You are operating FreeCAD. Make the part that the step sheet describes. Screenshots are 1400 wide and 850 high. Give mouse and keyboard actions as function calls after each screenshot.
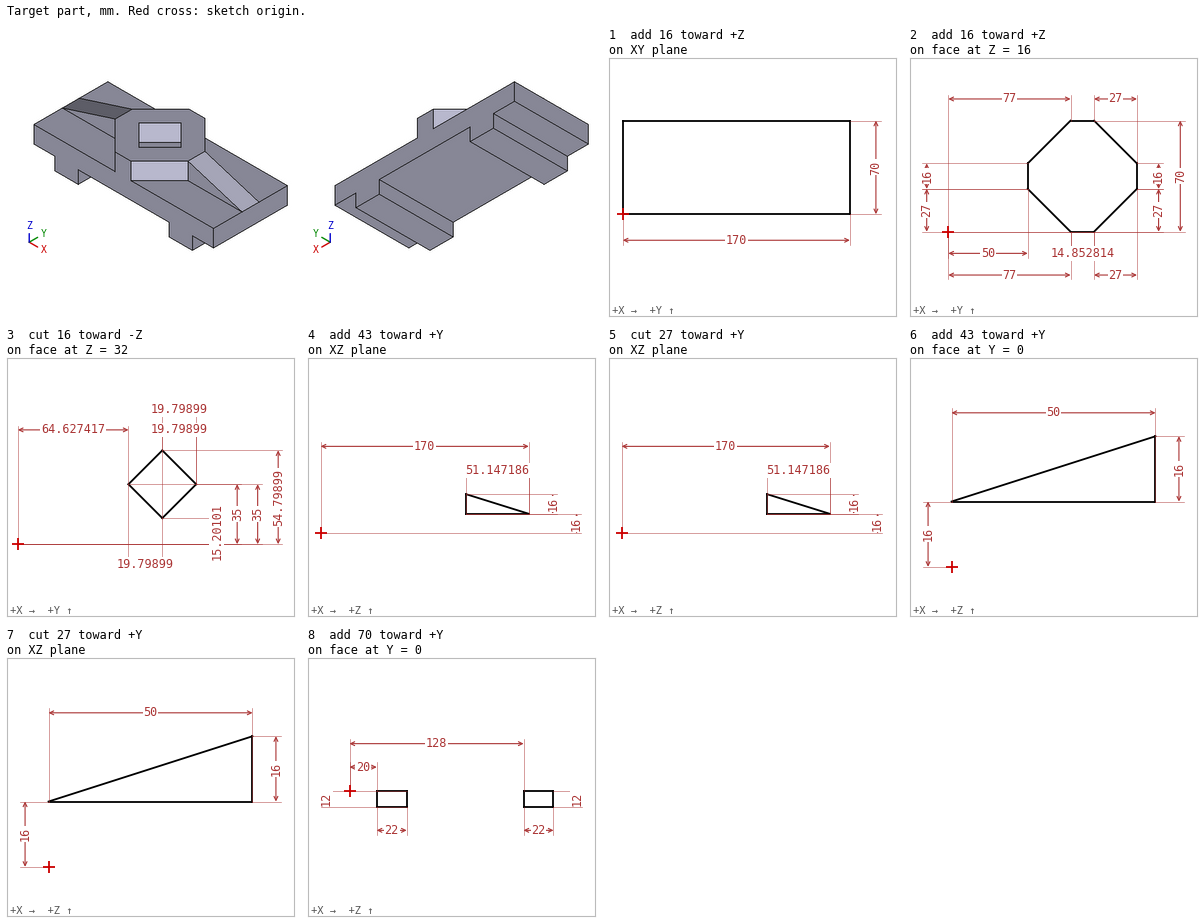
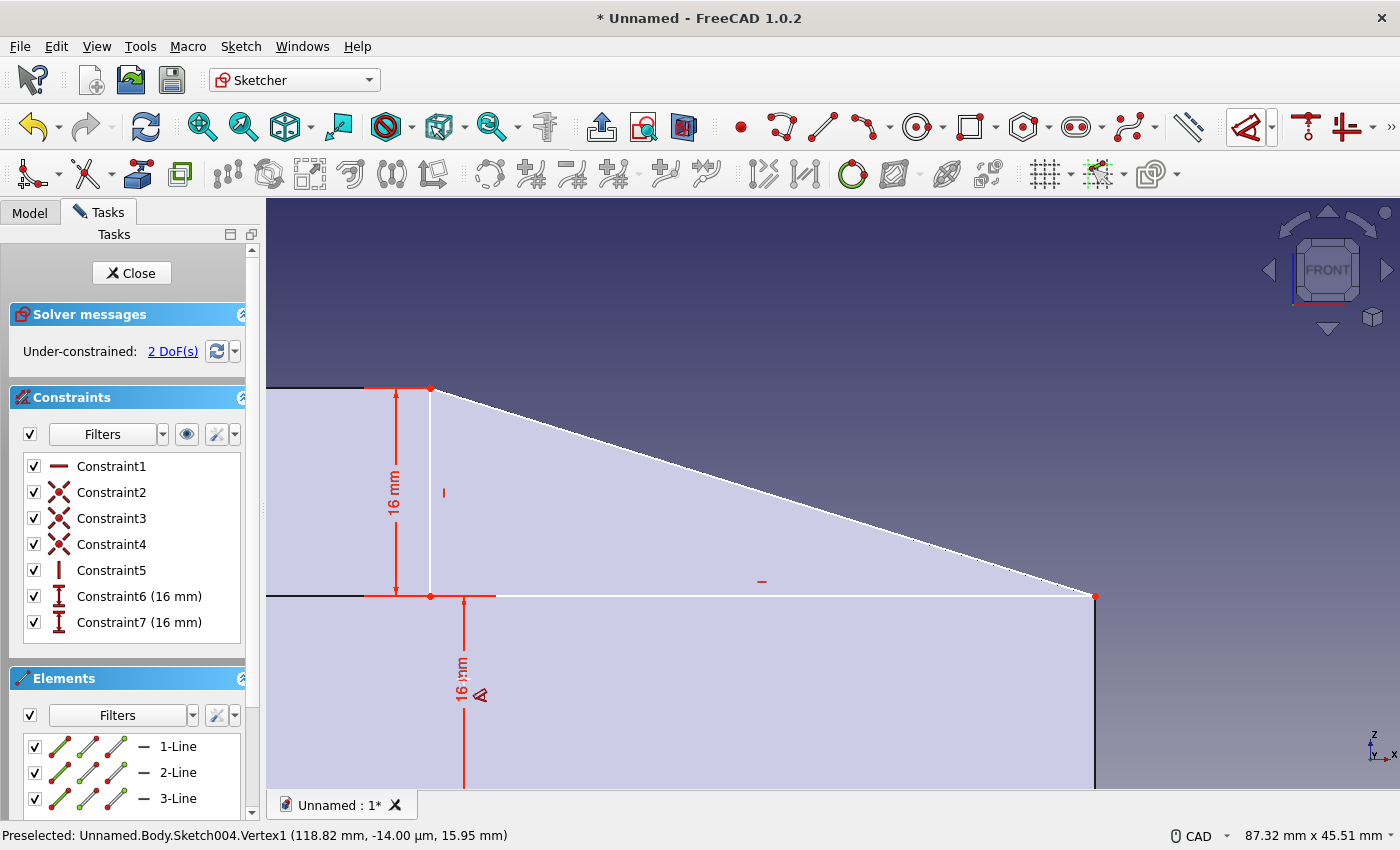
click(1095, 596)
click(695, 562)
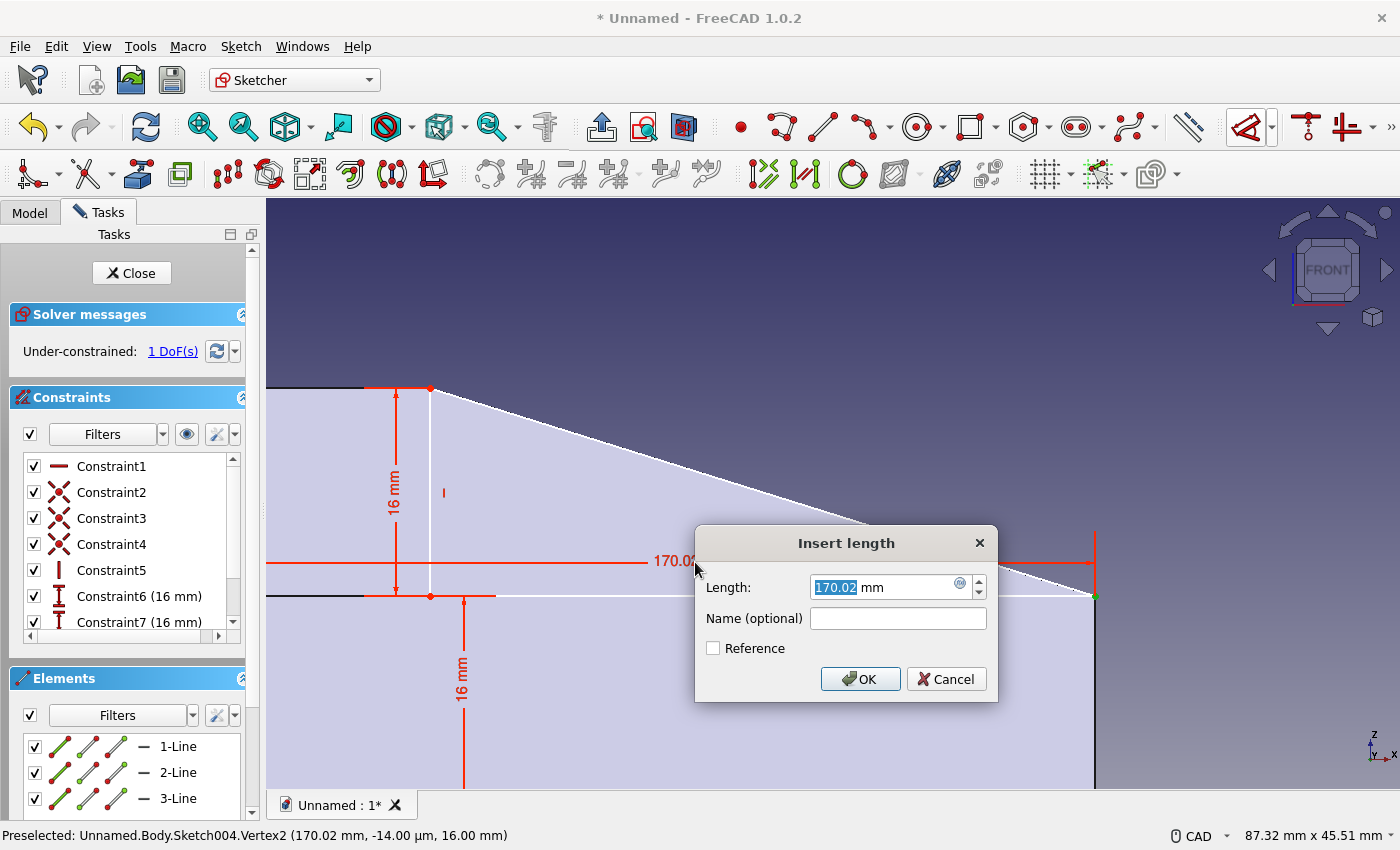
text(170)
key(Return)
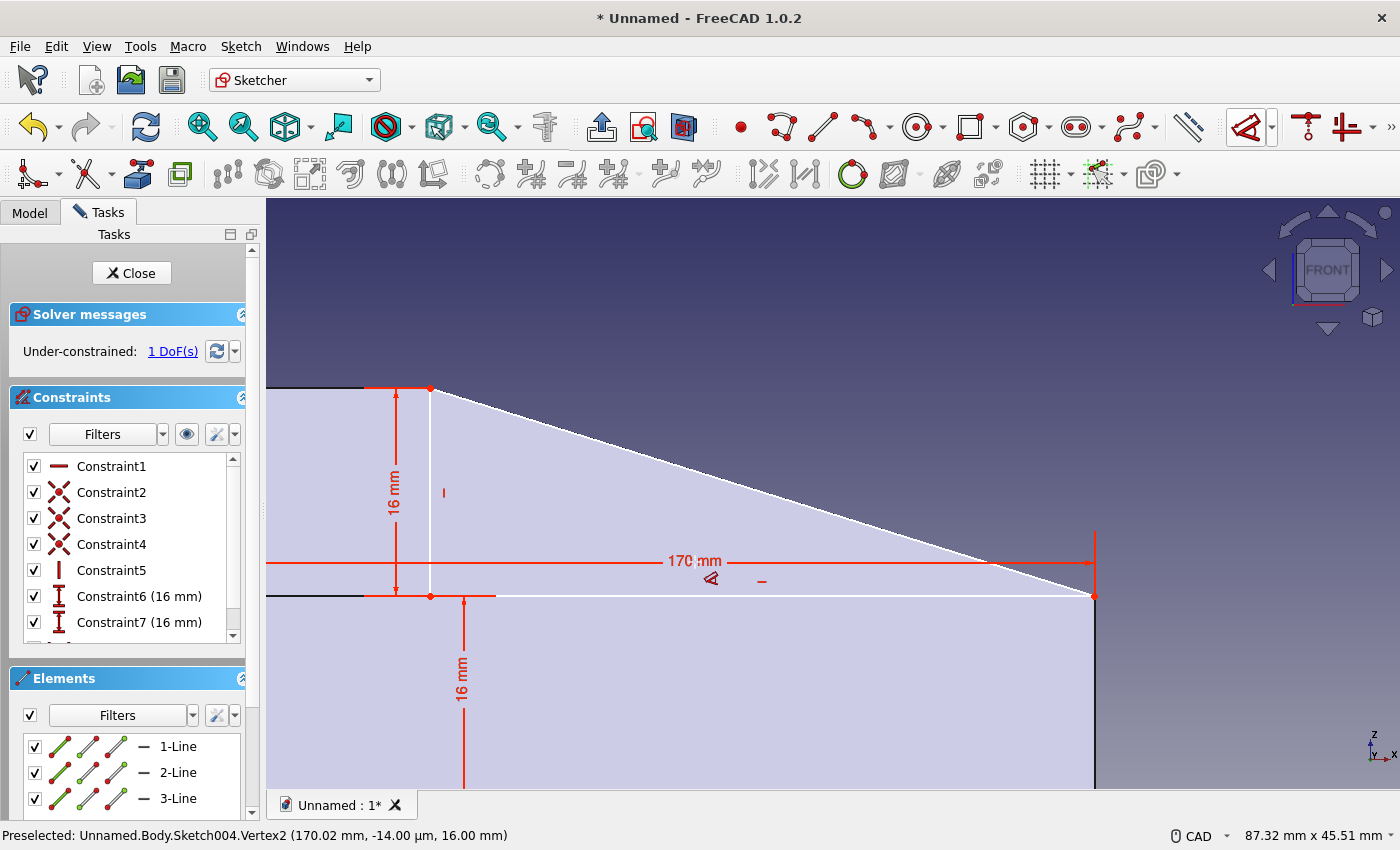
click(629, 596)
click(762, 630)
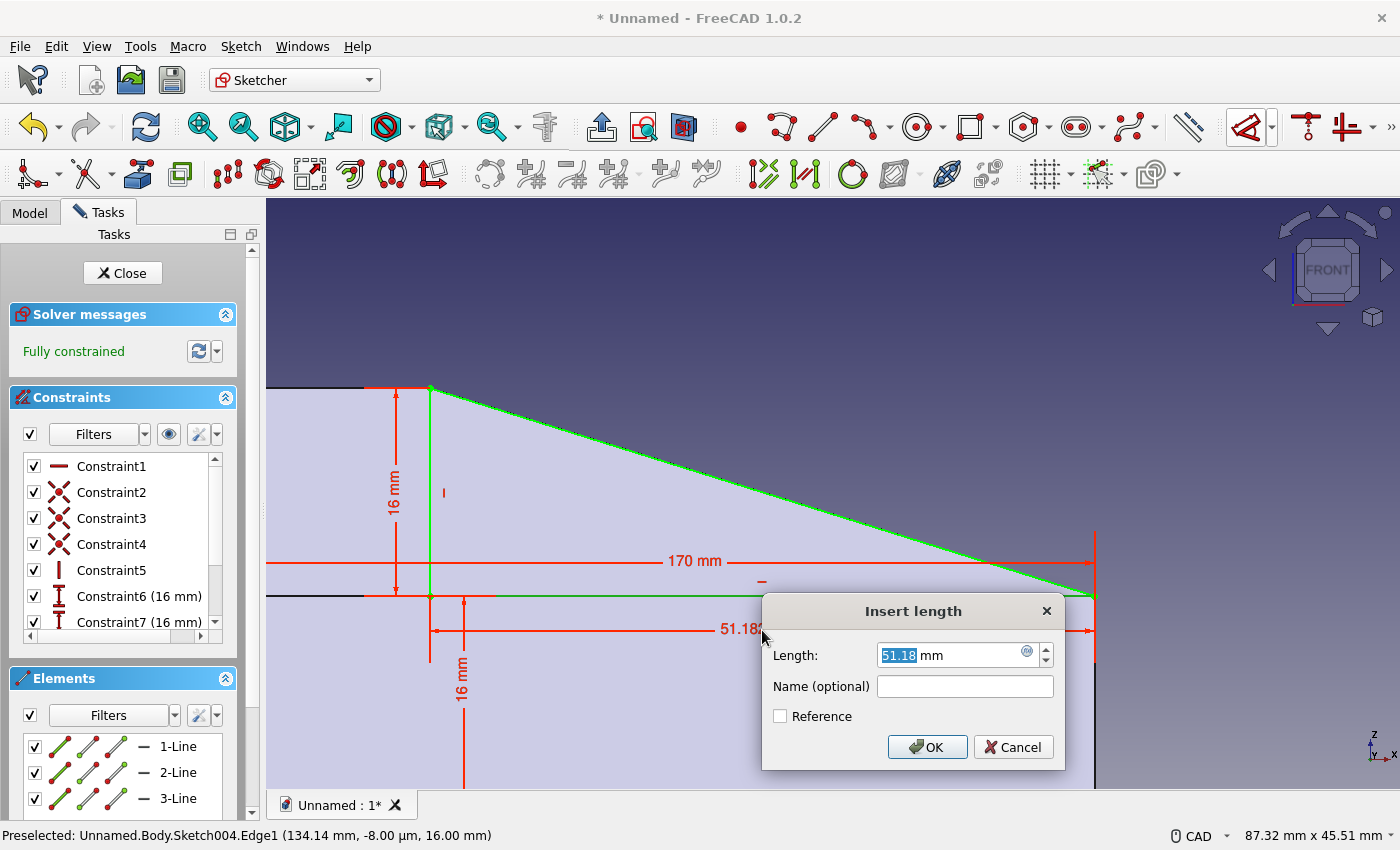
text(51.147186)
key(Return)
key(Escape)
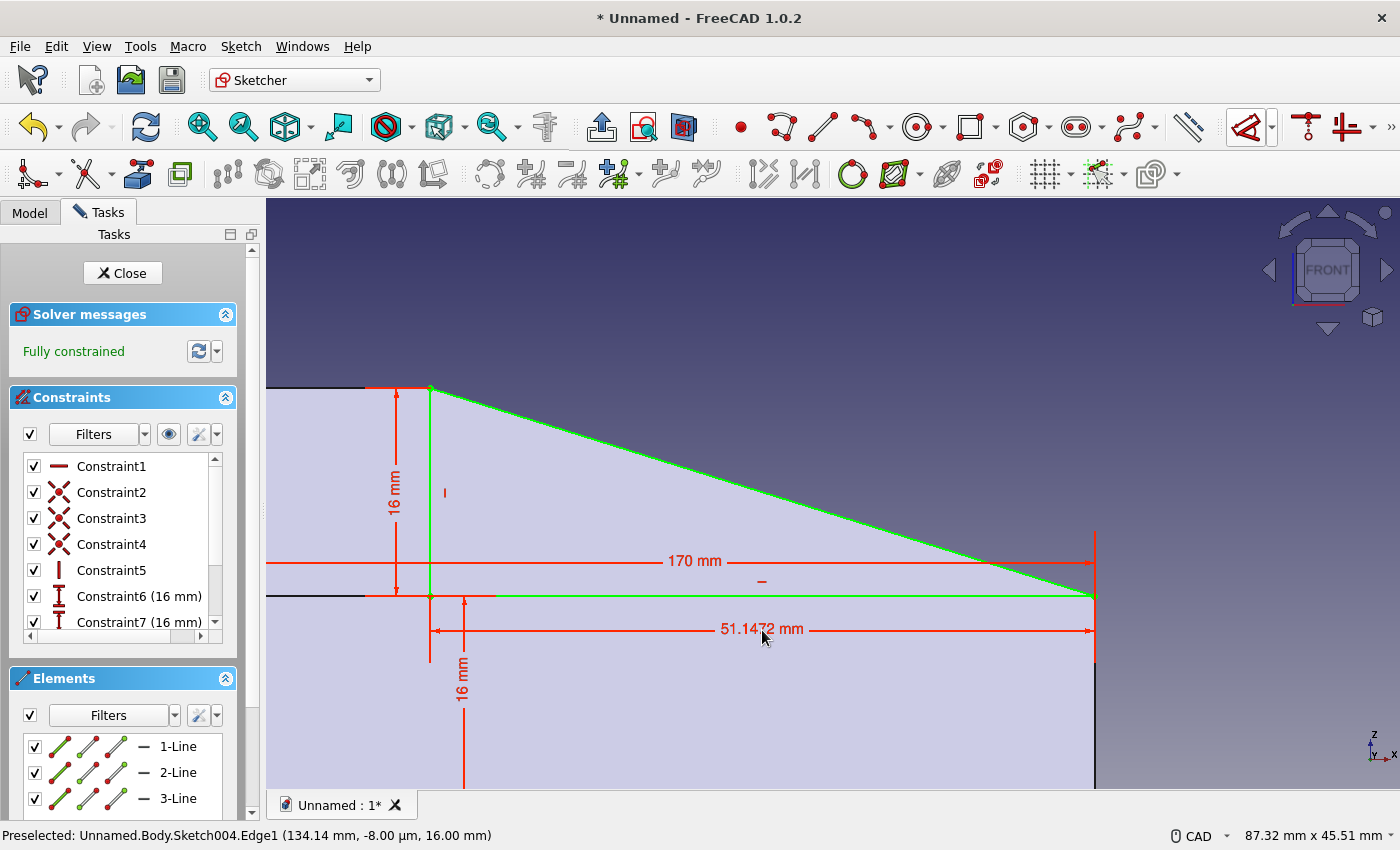
click(123, 273)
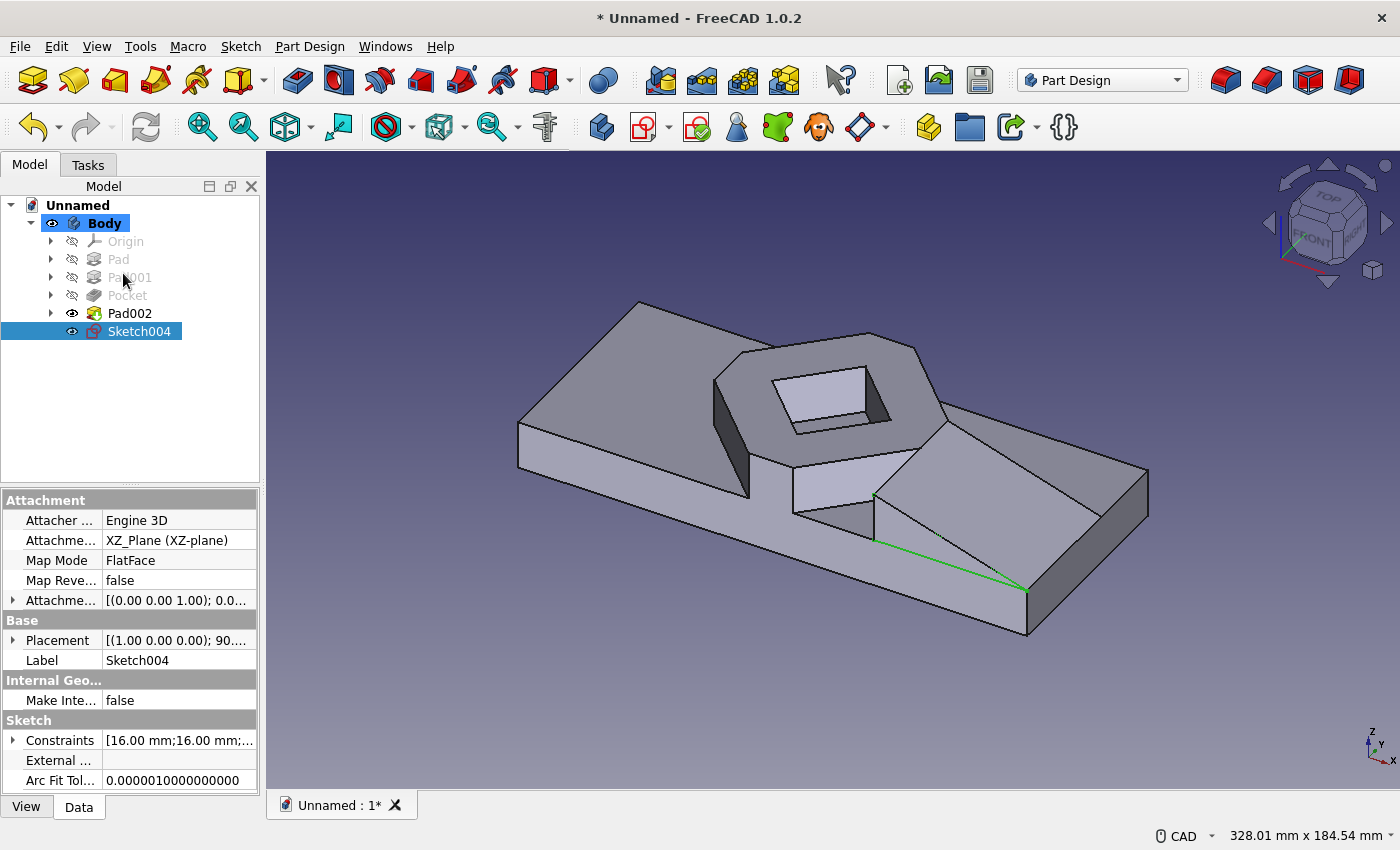
click(298, 80)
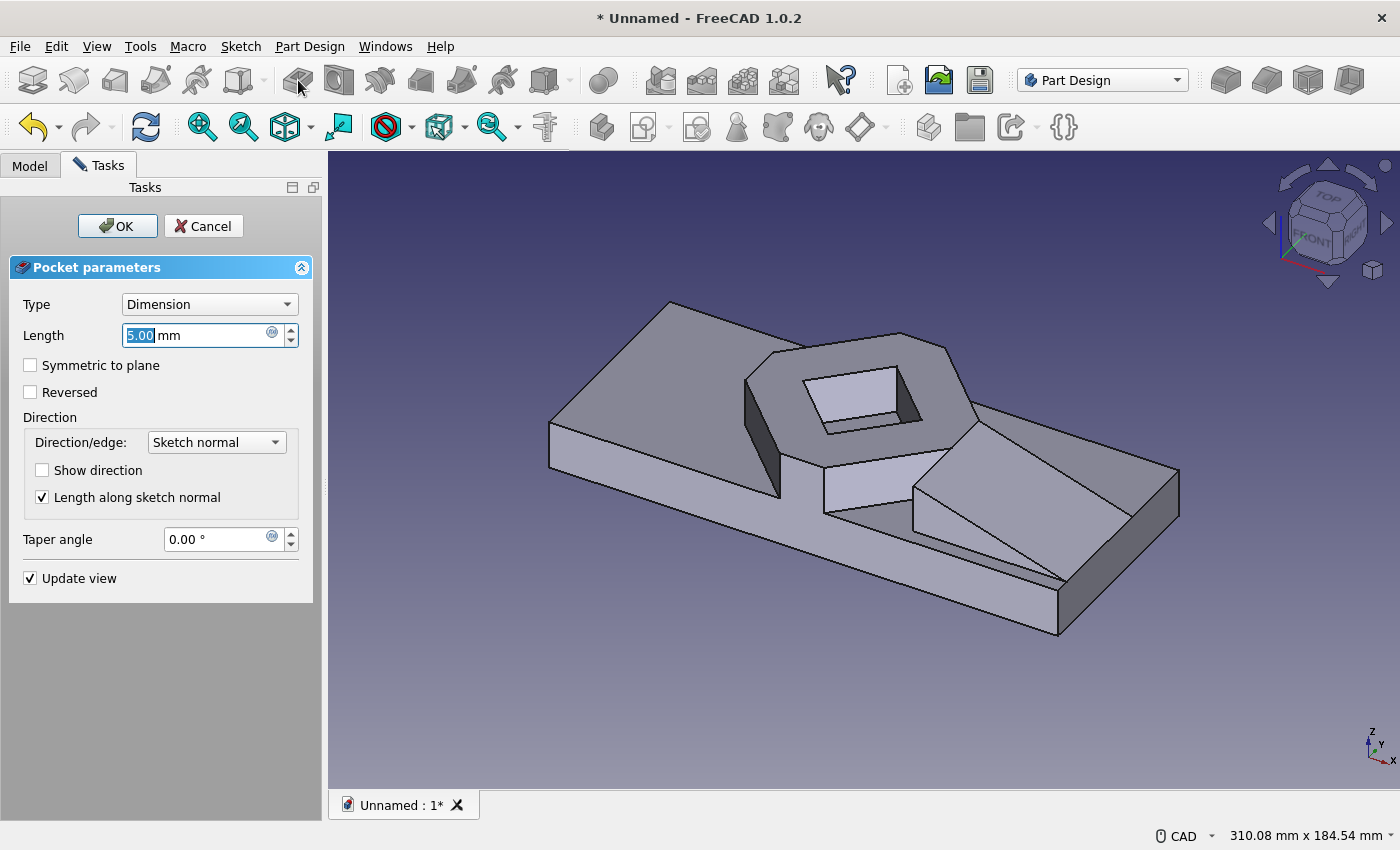
text(27)
key(Tab)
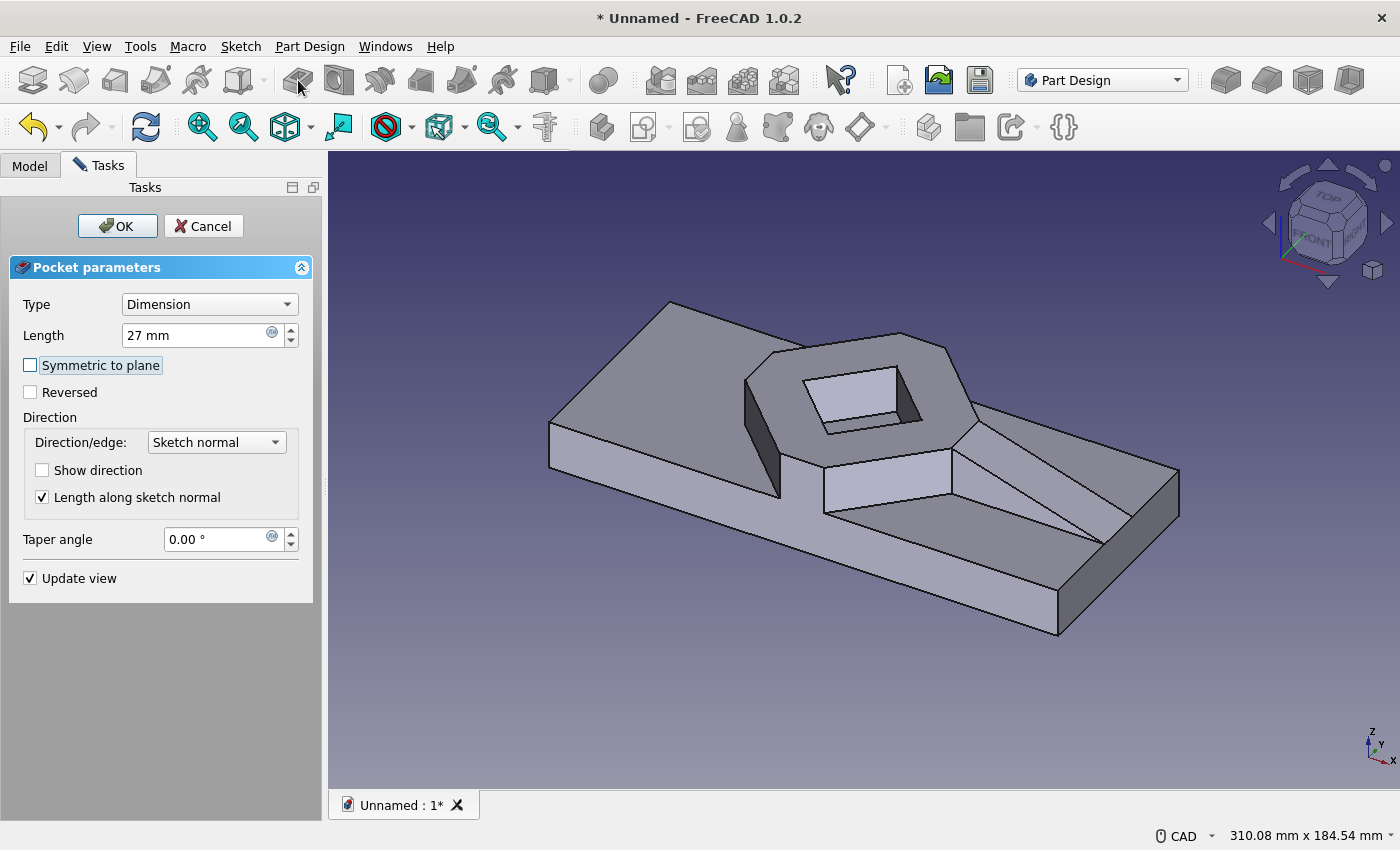
click(118, 226)